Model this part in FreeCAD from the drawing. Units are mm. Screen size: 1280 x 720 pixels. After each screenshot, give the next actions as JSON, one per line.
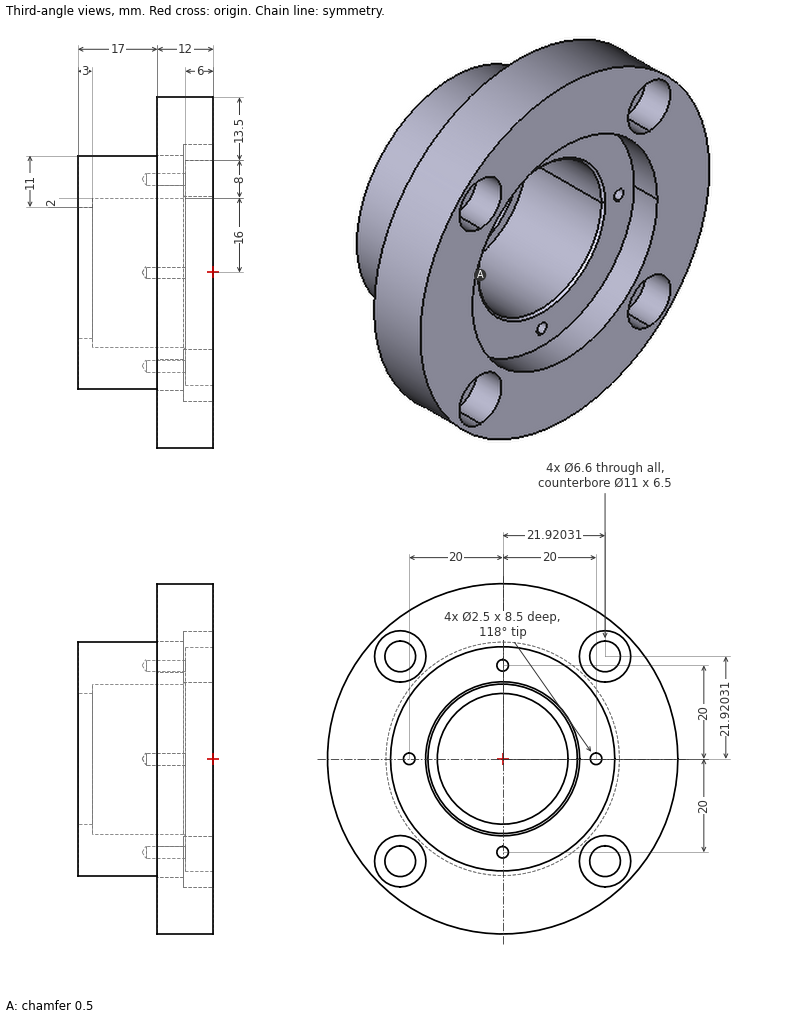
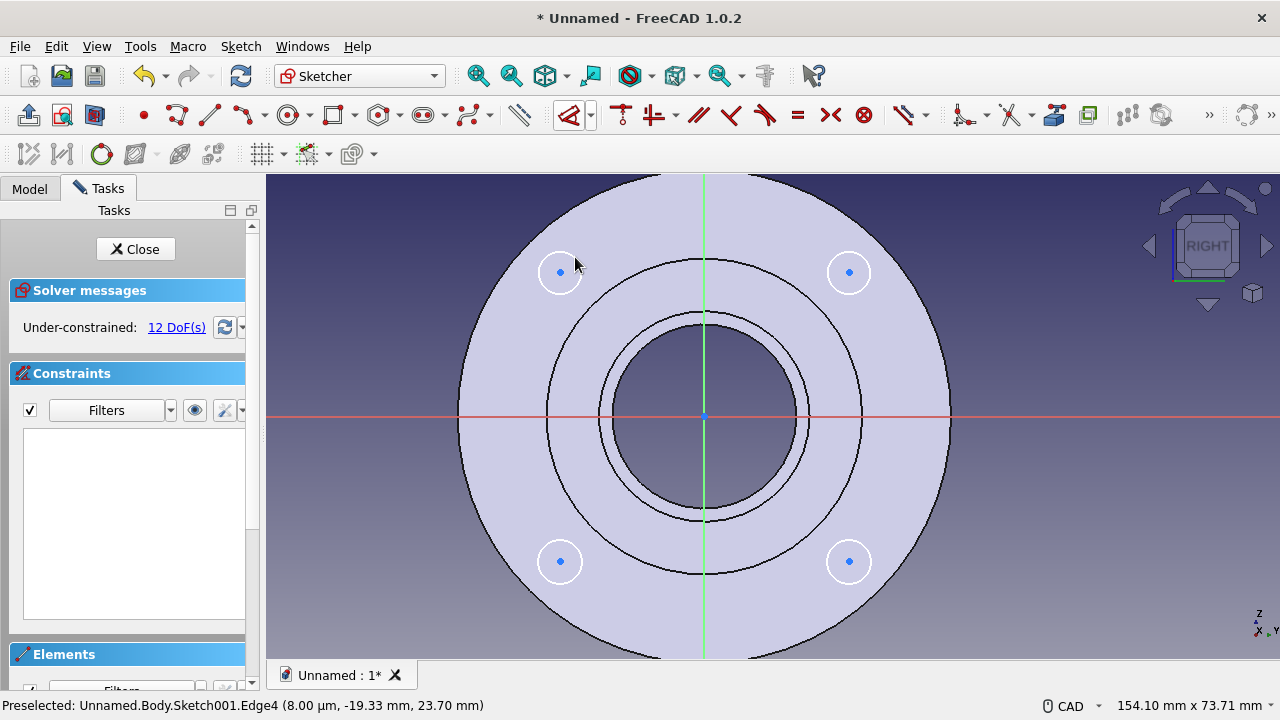
{"action": "left_click", "coordinate": [864, 258]}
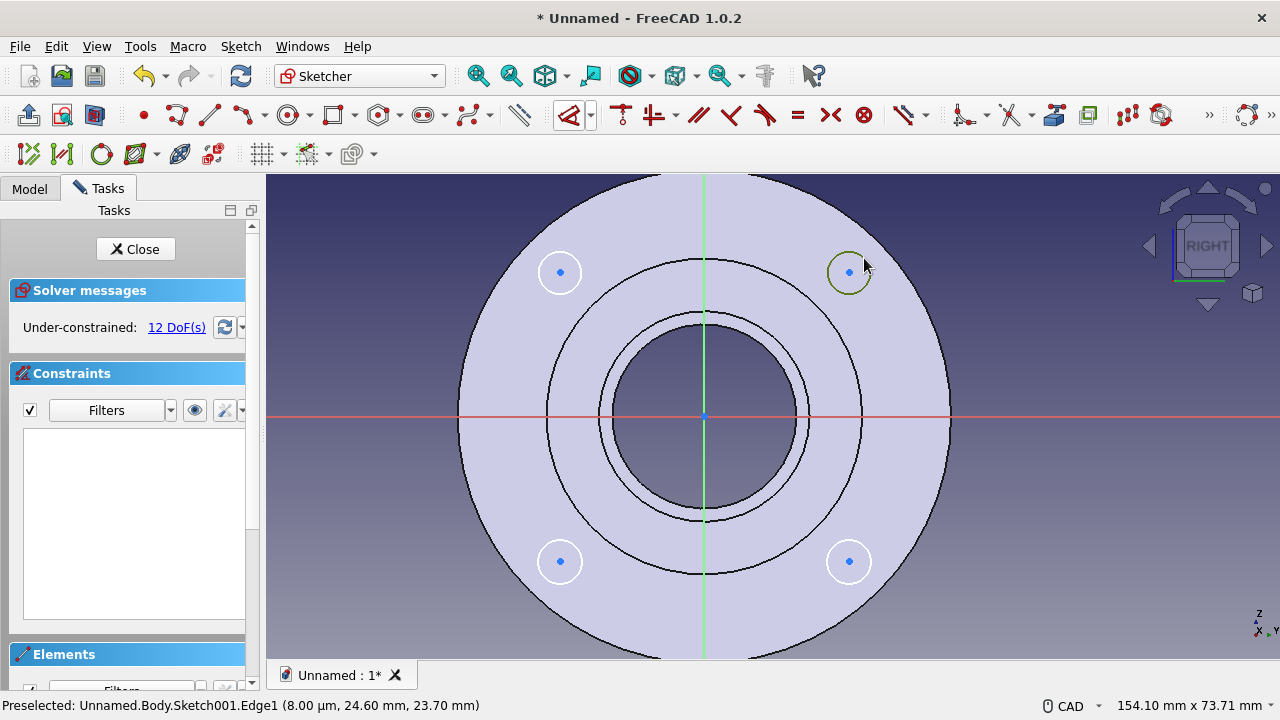
{"action": "left_click", "coordinate": [864, 546]}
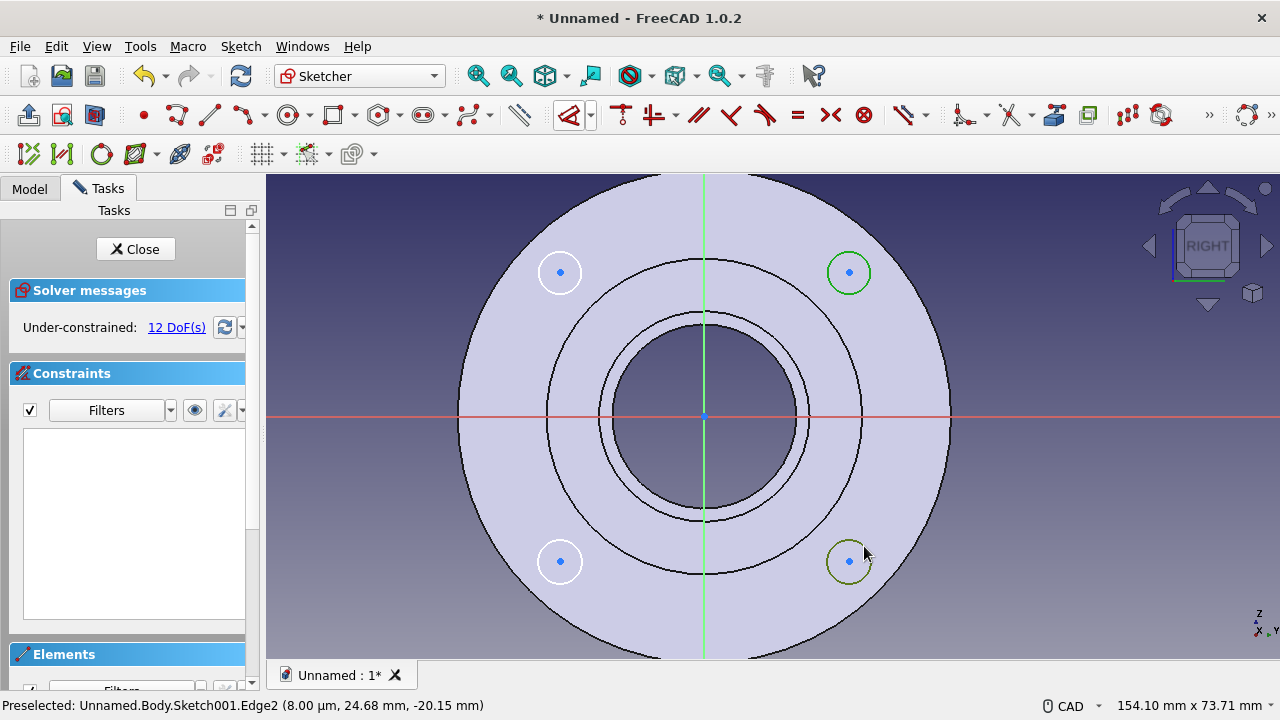
{"action": "left_click", "coordinate": [575, 546]}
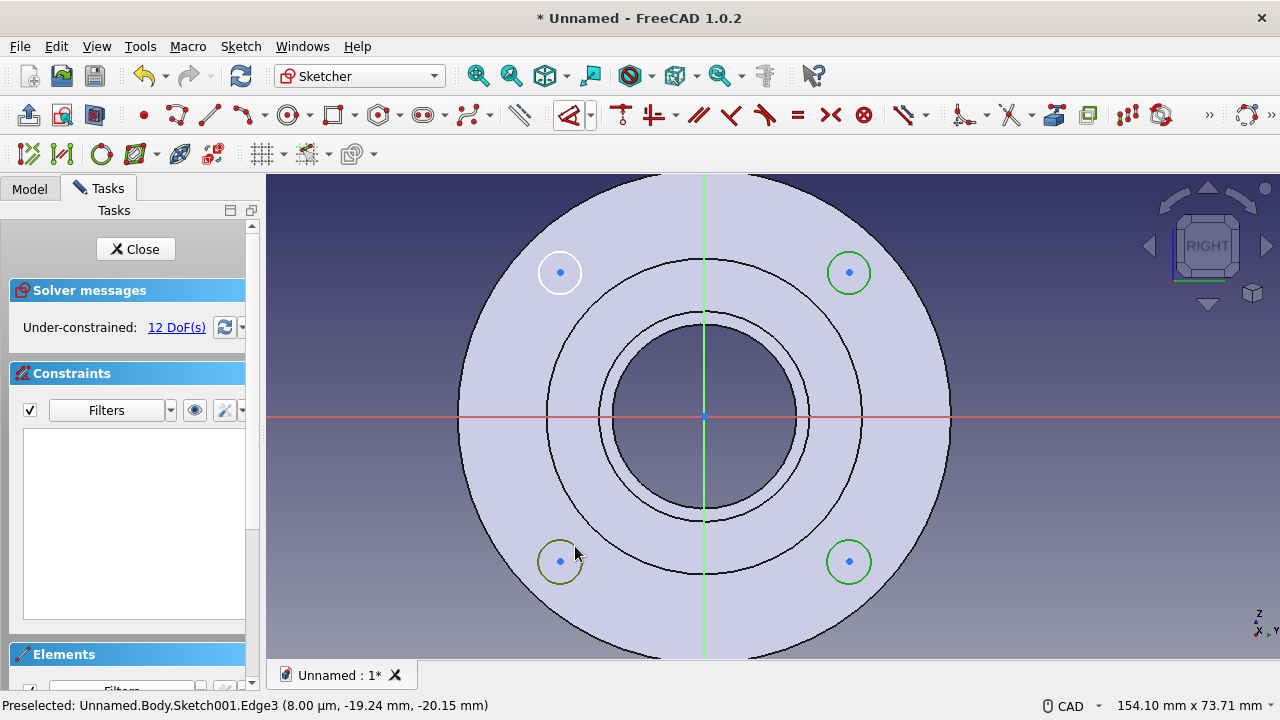
{"action": "left_click", "coordinate": [575, 258]}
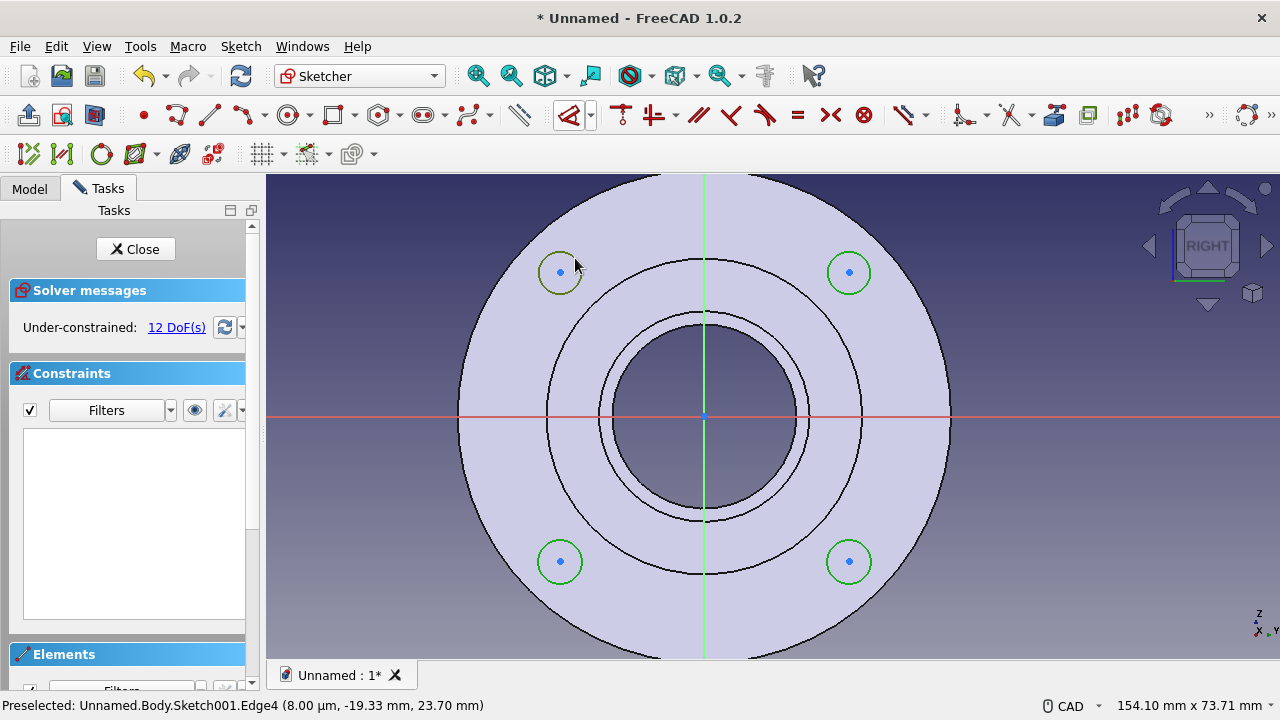
{"action": "key", "text": "e"}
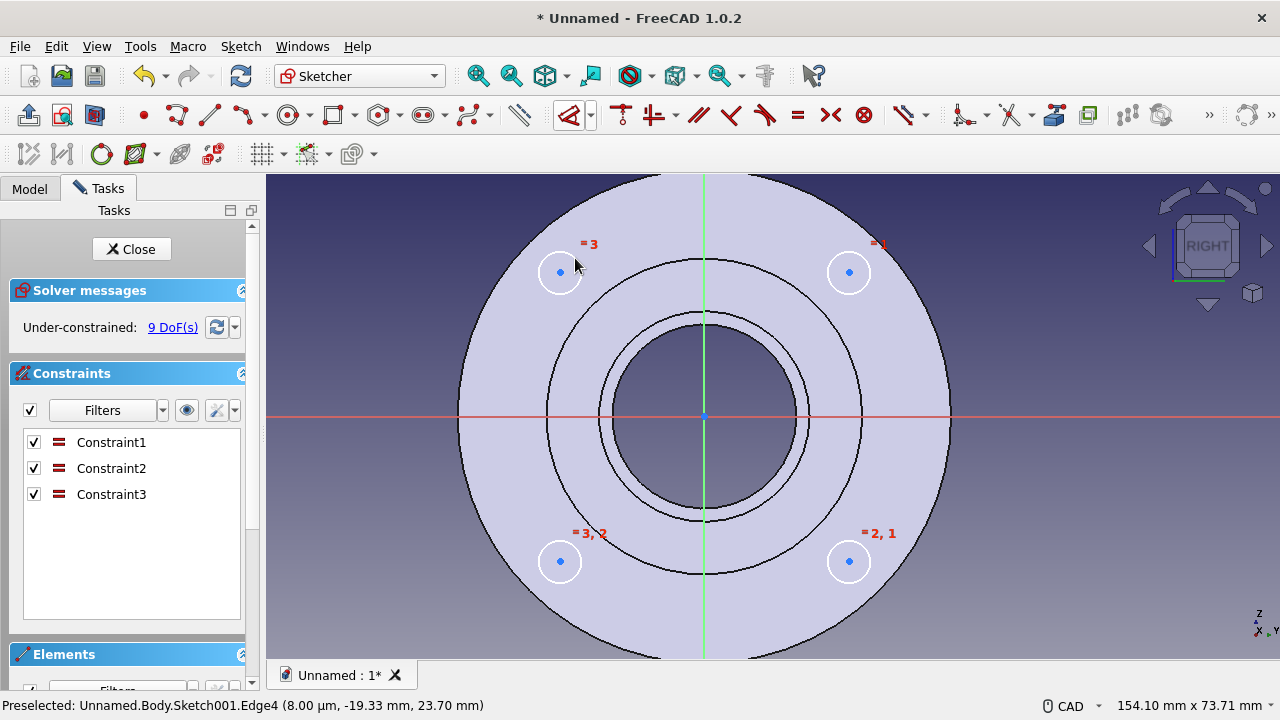
{"action": "left_click", "coordinate": [849, 273]}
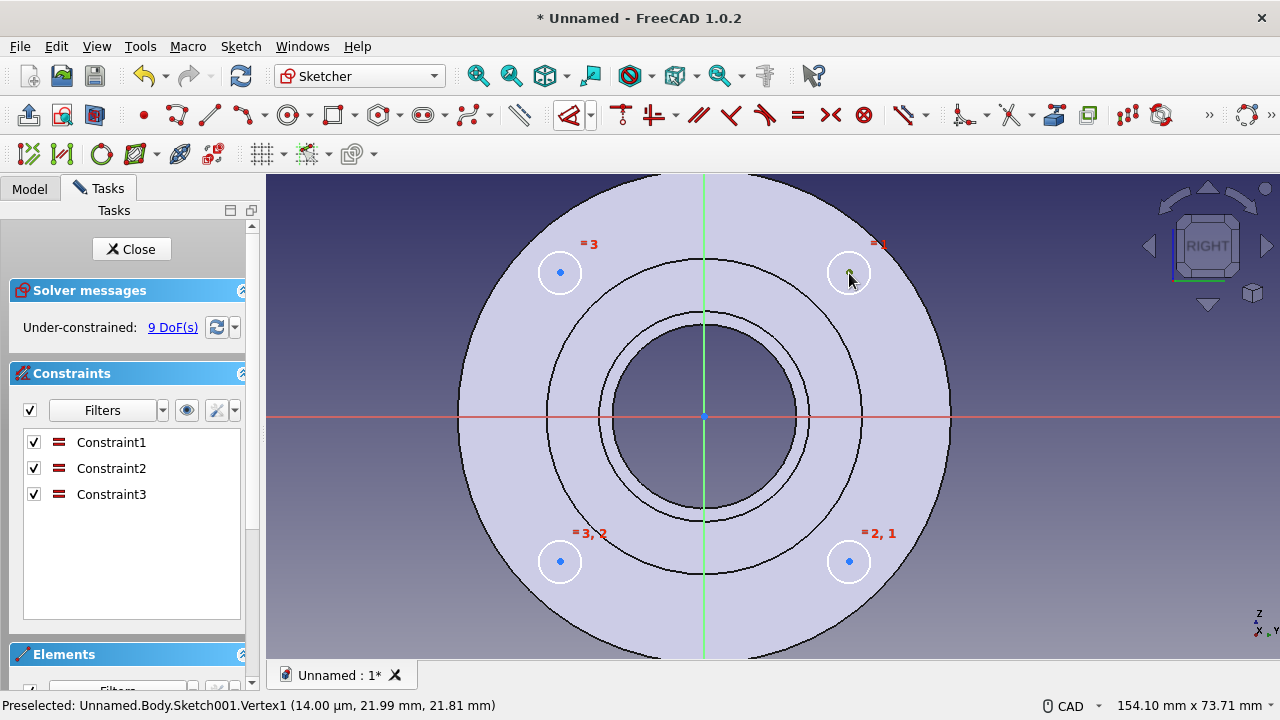
{"action": "left_click", "coordinate": [849, 562]}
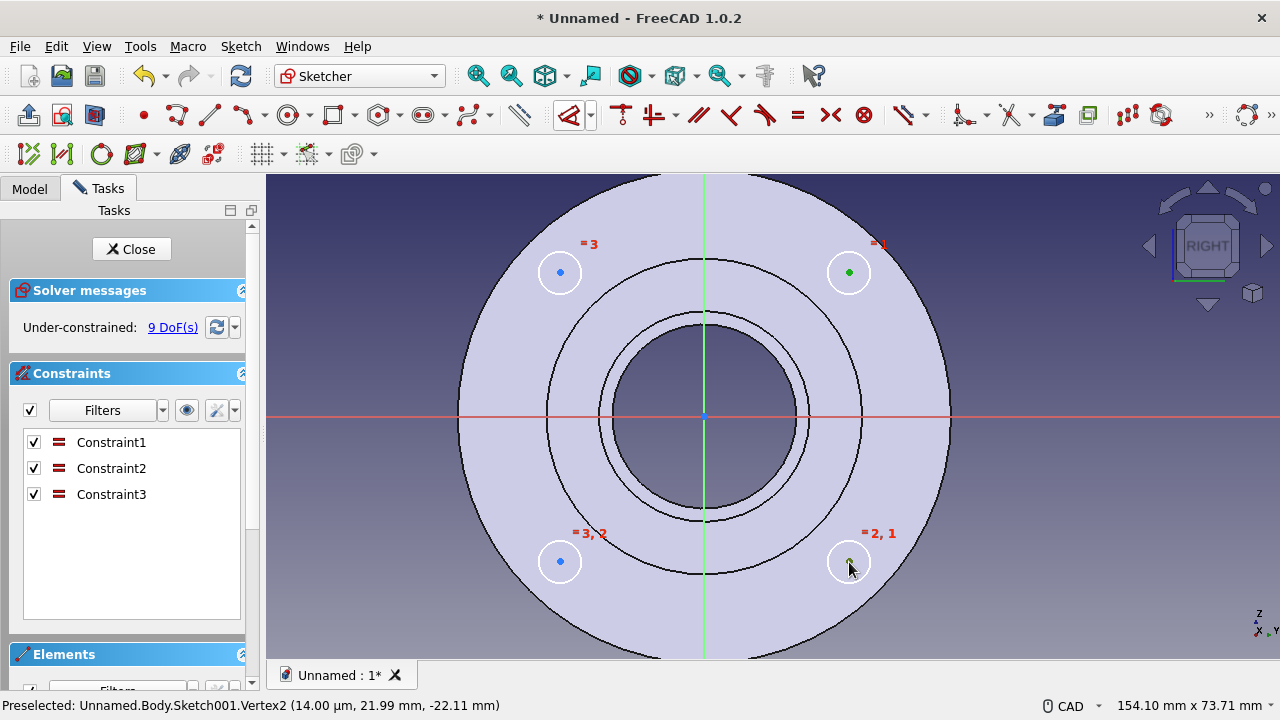
{"action": "left_click", "coordinate": [353, 416]}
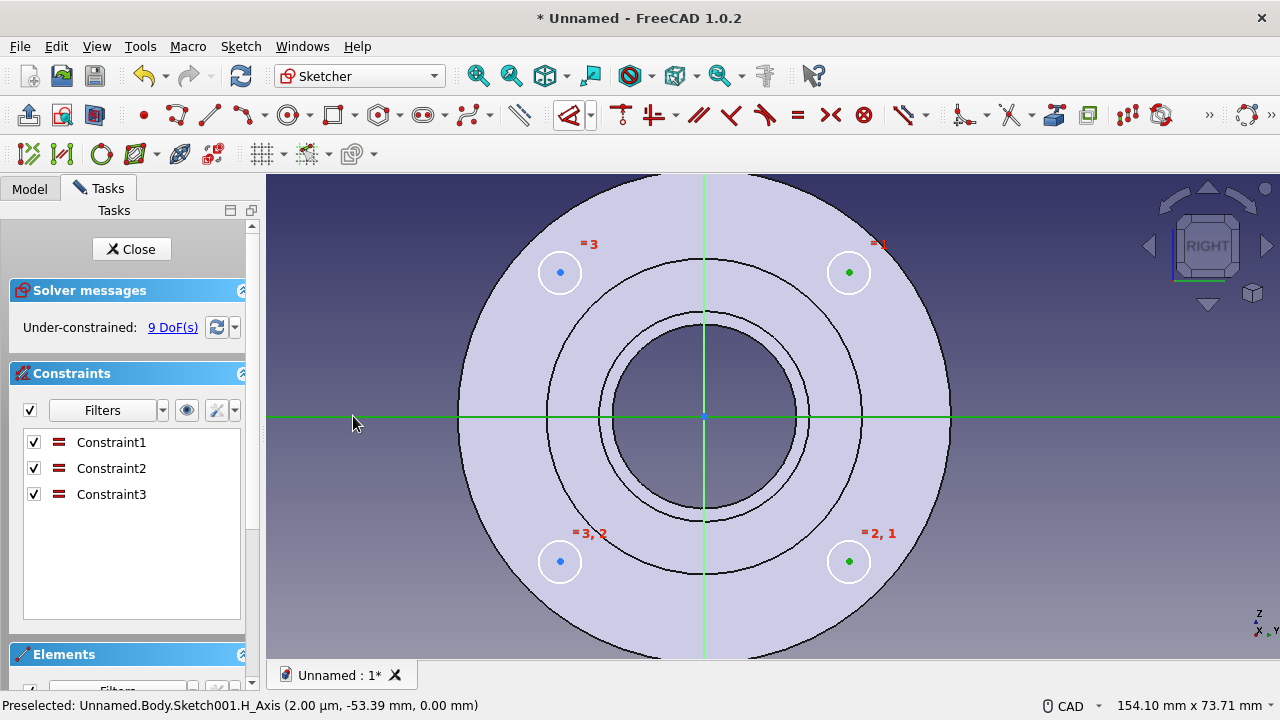
{"action": "key", "text": "s"}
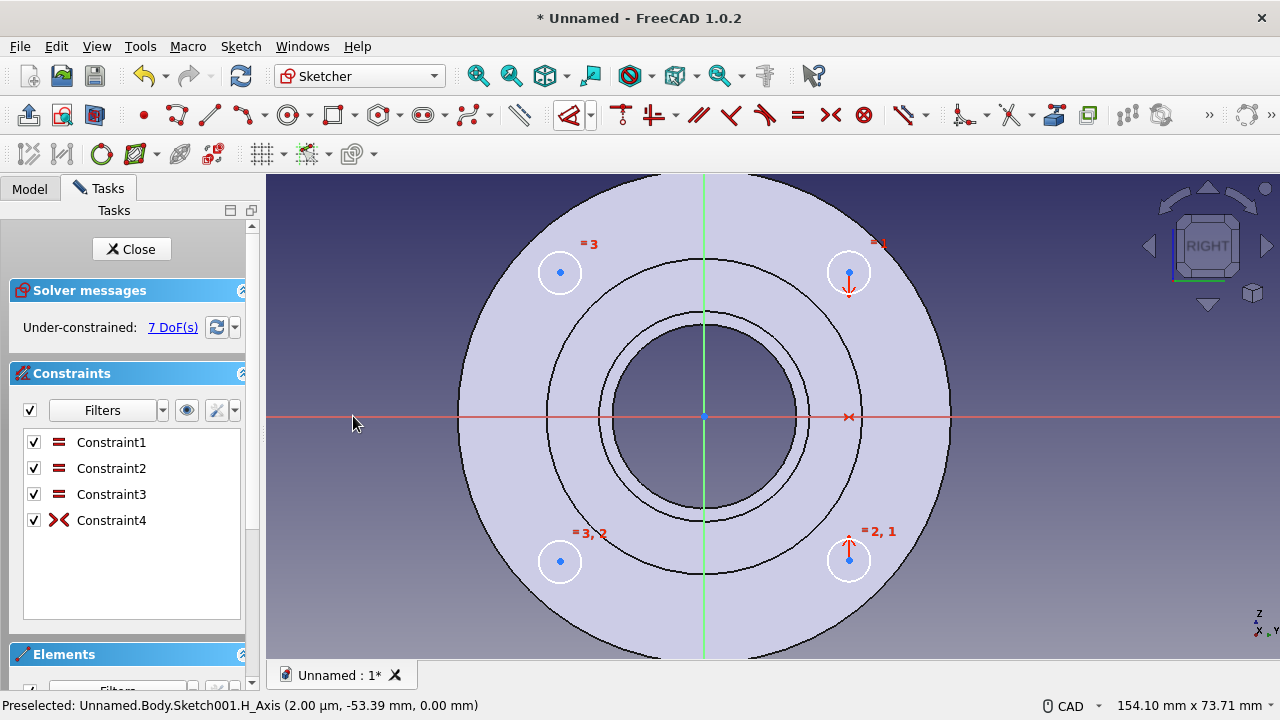
{"action": "left_click", "coordinate": [849, 560]}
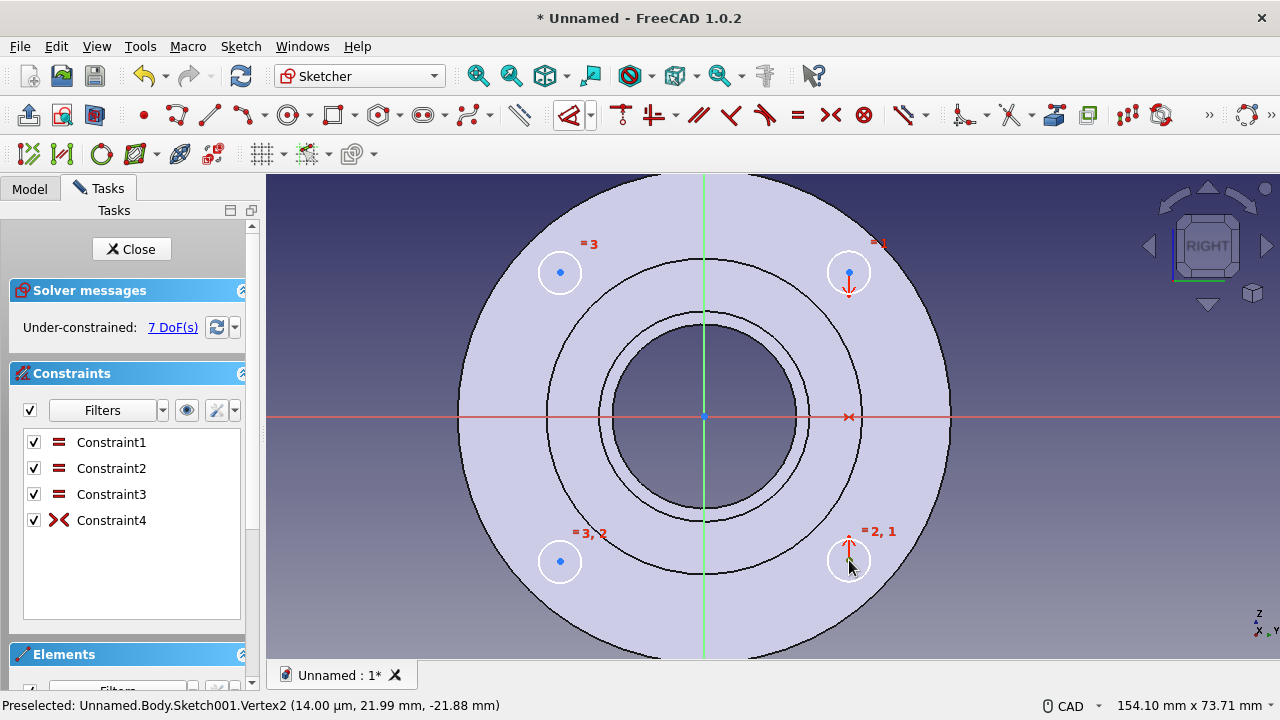
{"action": "left_click", "coordinate": [560, 562]}